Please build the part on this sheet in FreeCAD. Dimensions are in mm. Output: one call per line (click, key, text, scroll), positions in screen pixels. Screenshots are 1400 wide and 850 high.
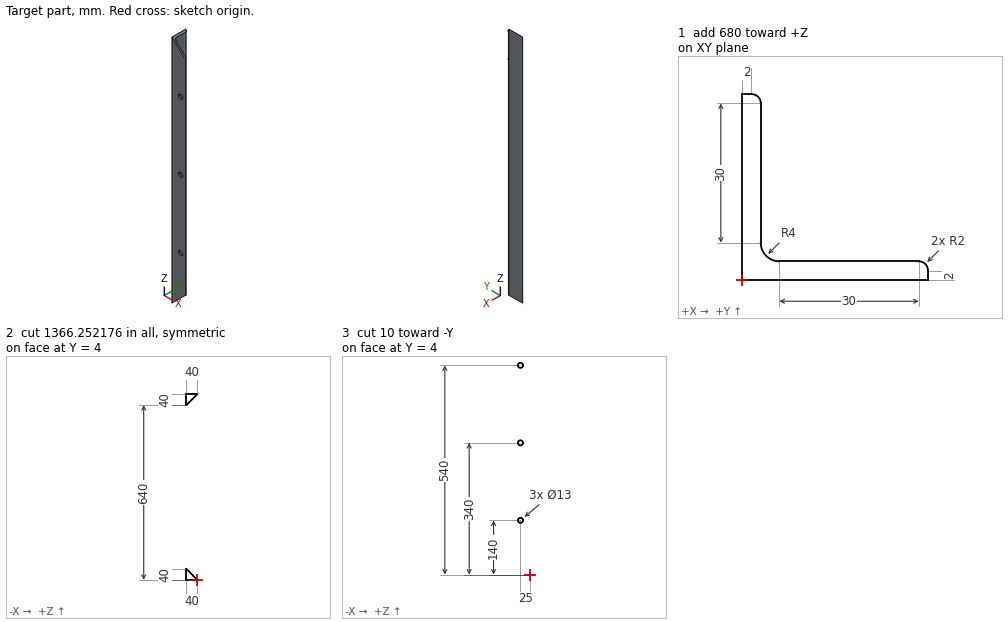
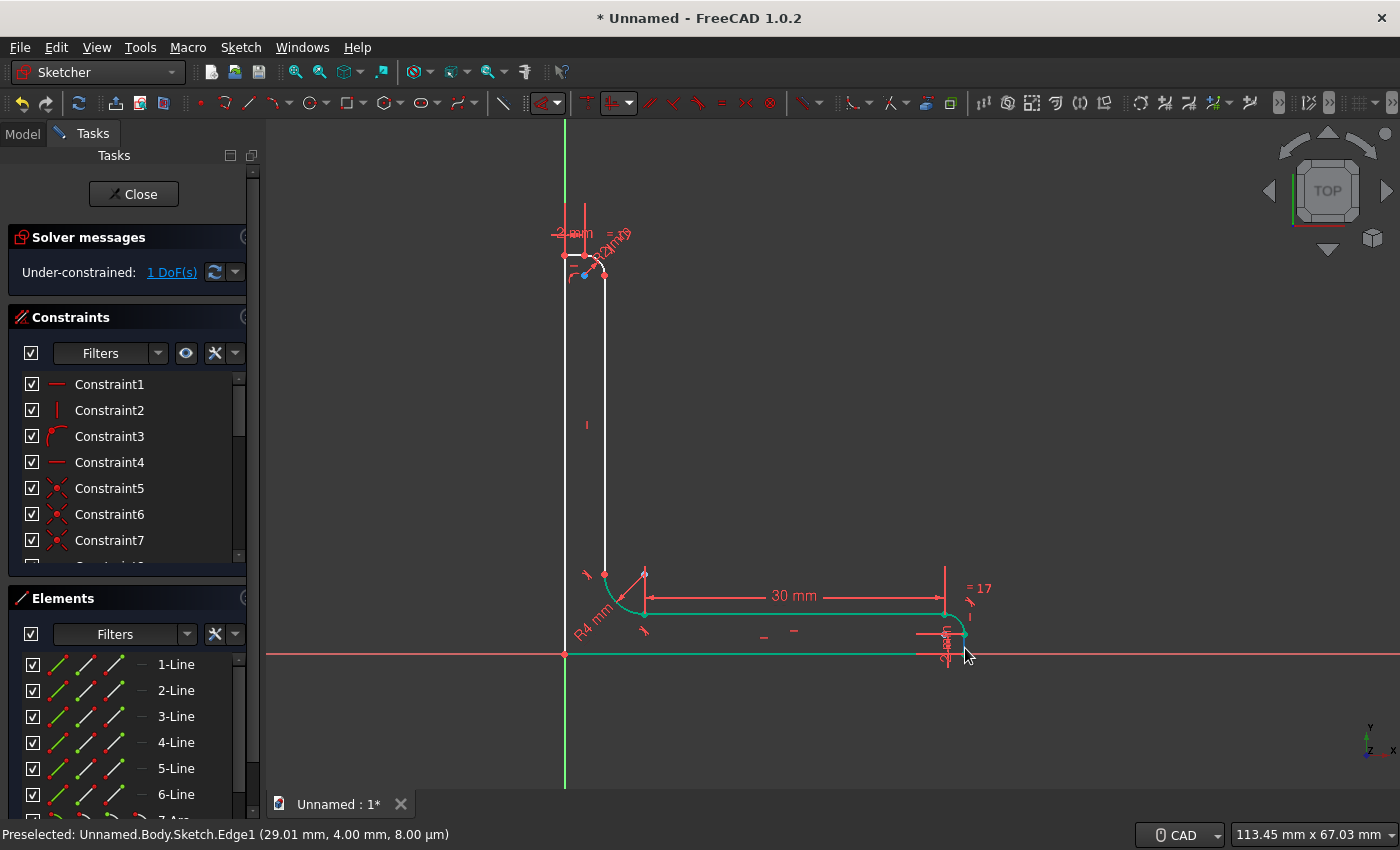
click(605, 484)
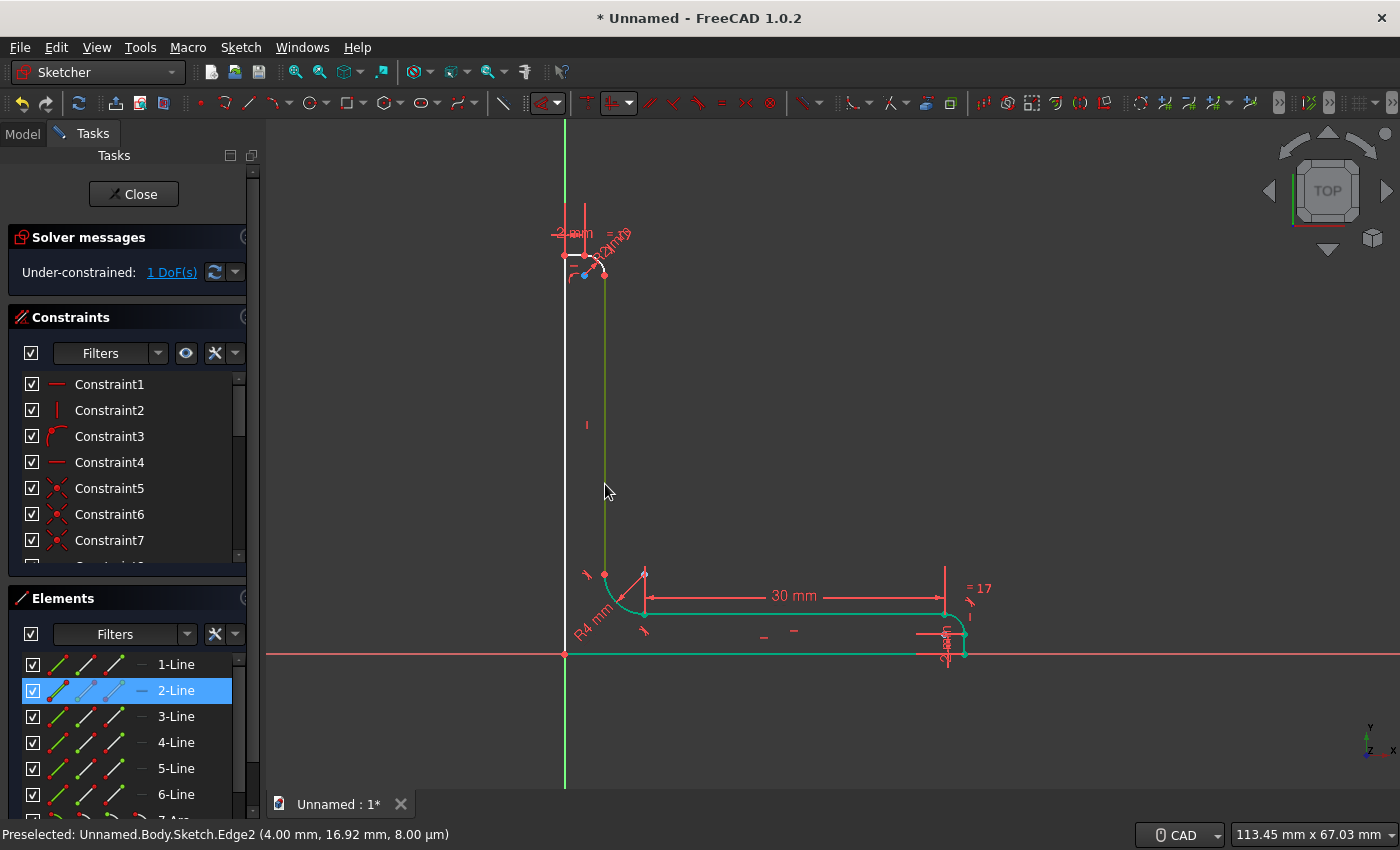
key(i)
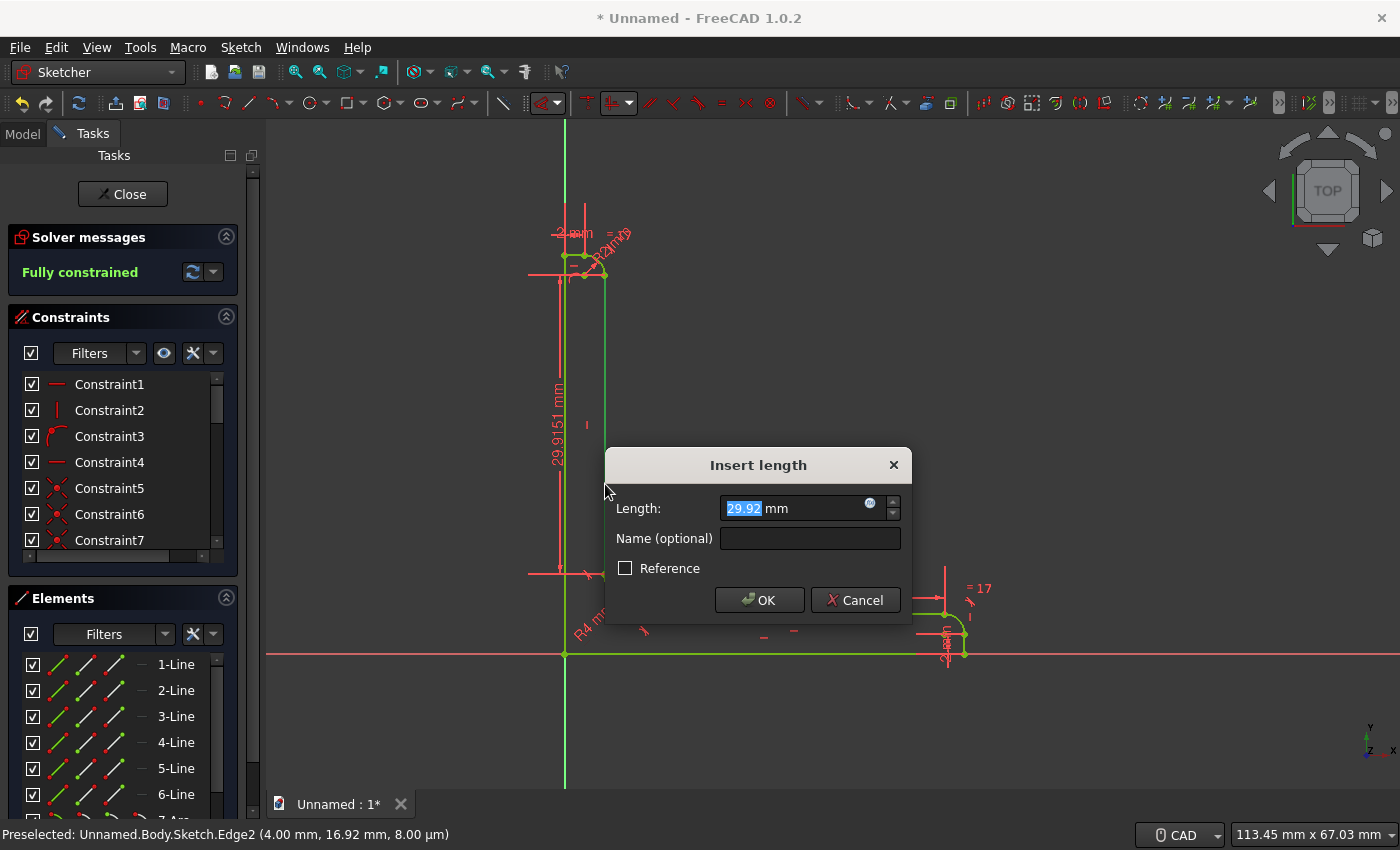
text(30)
key(Return)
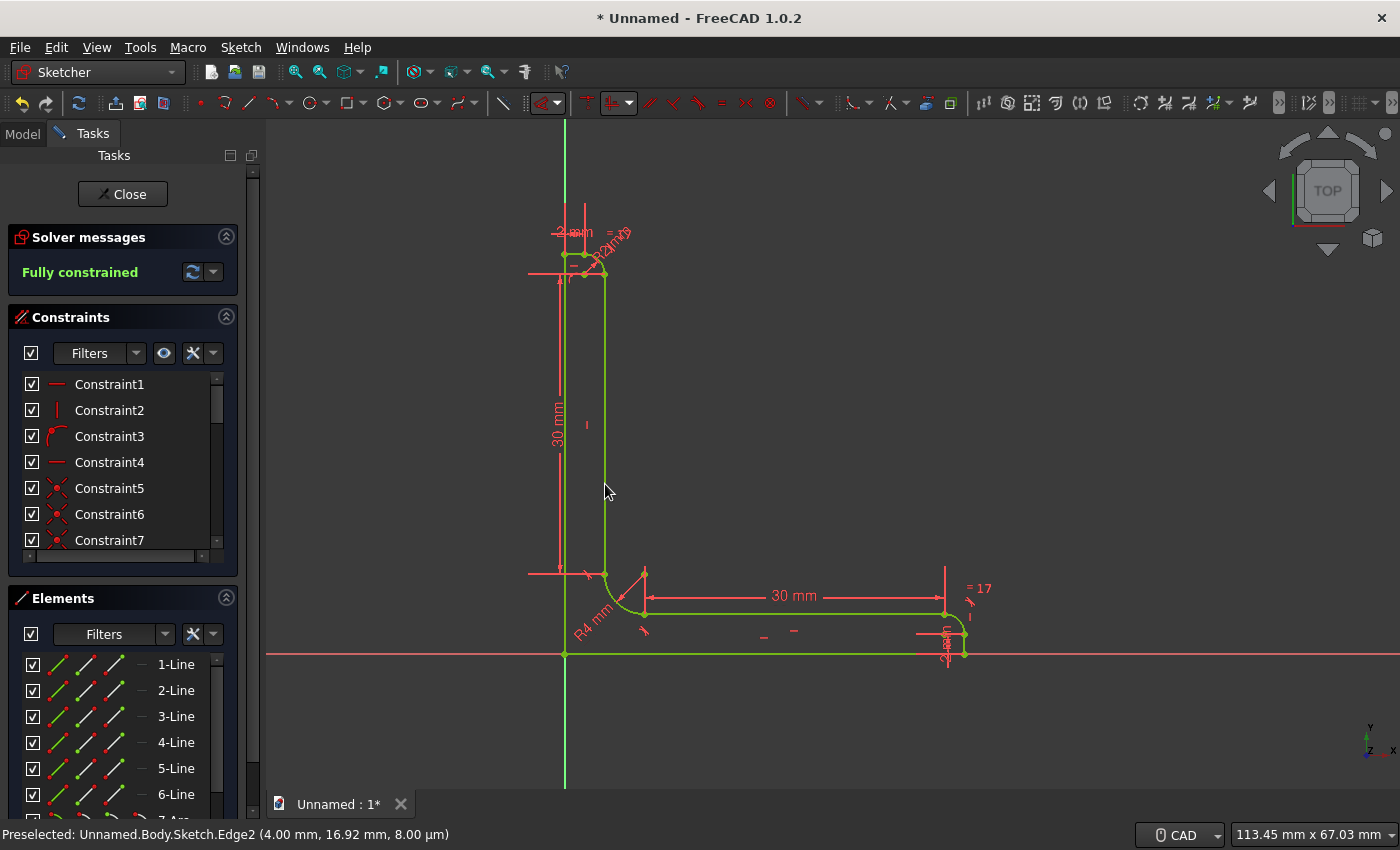
click(123, 194)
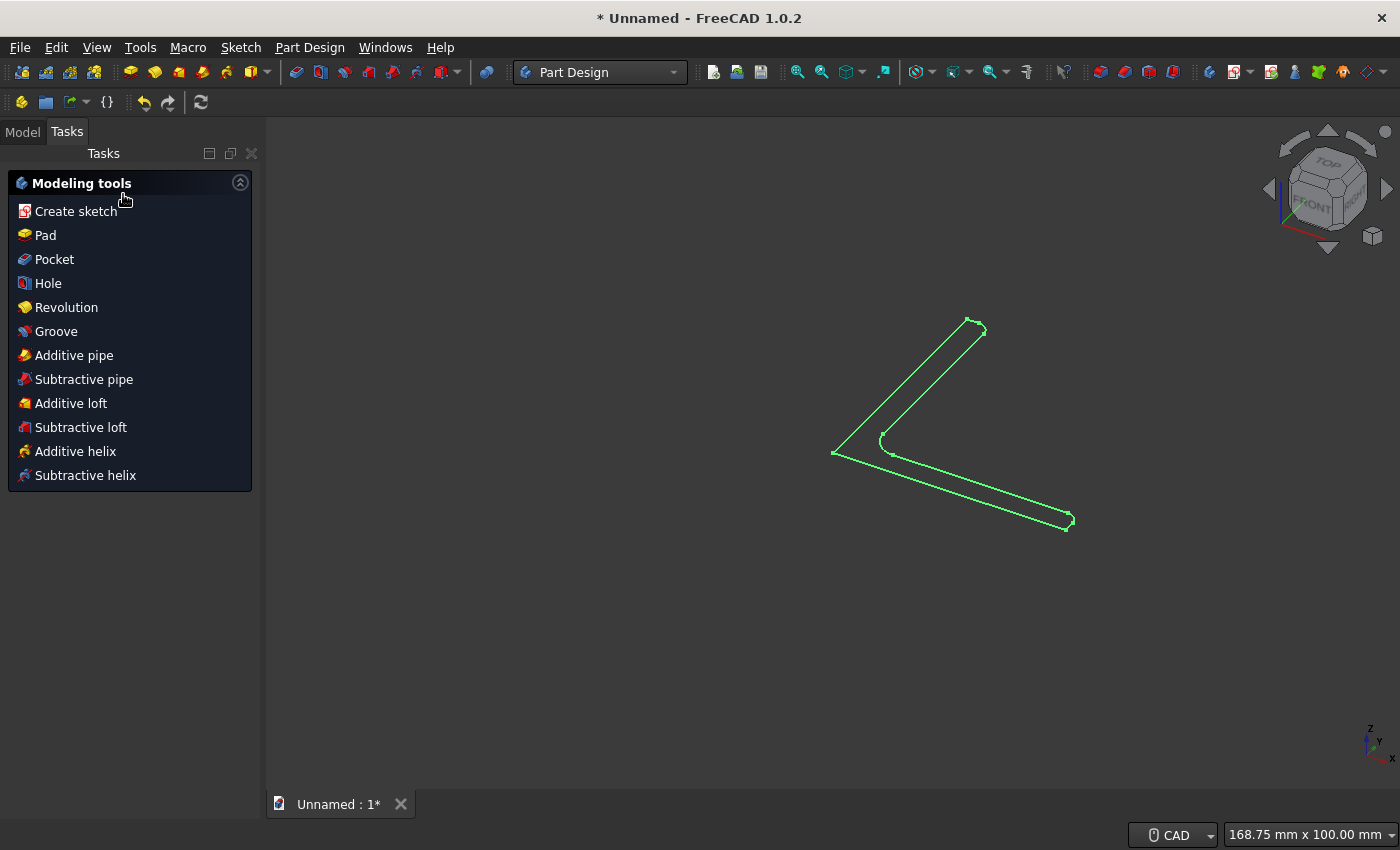
click(132, 72)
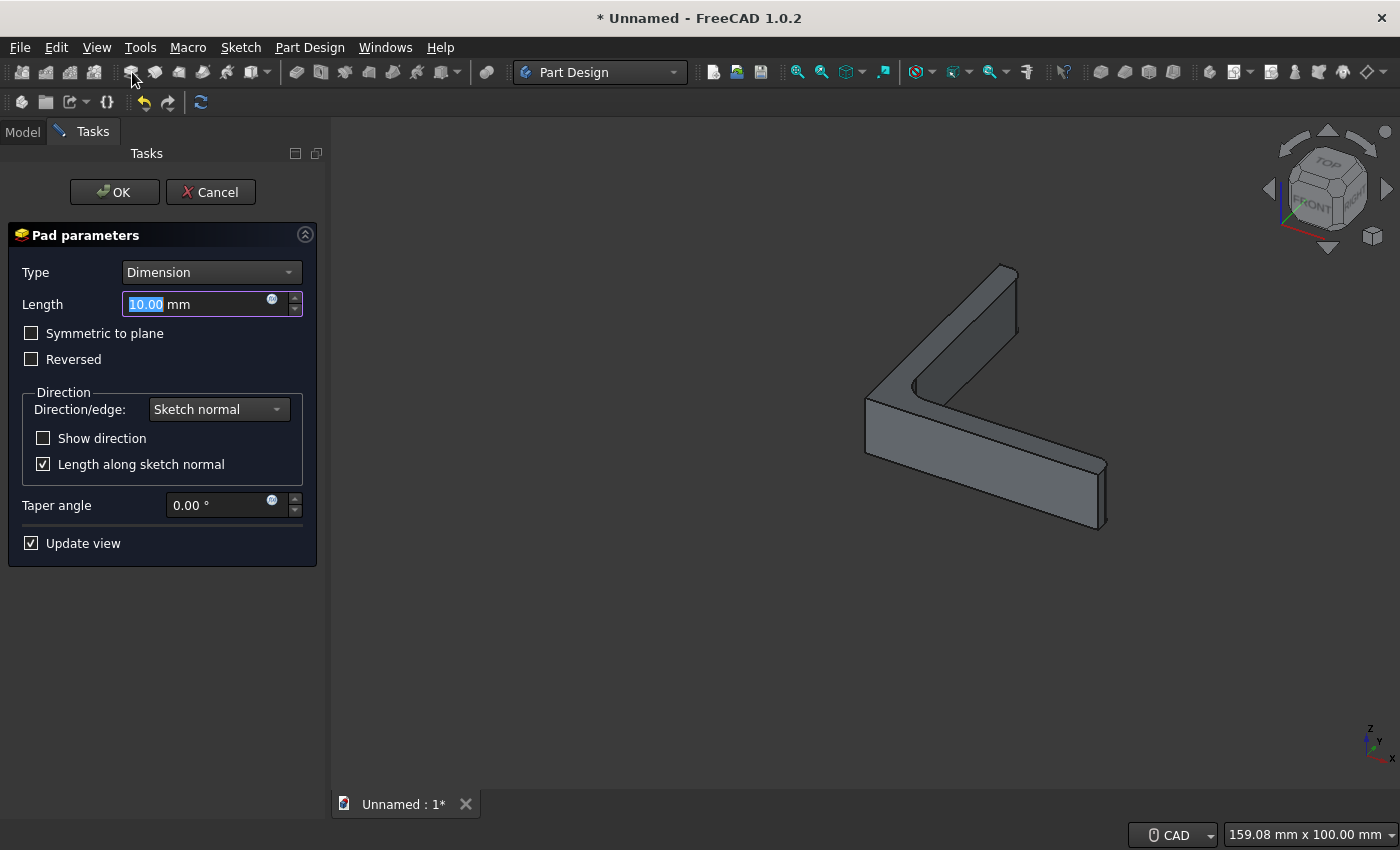
text(680)
key(Tab)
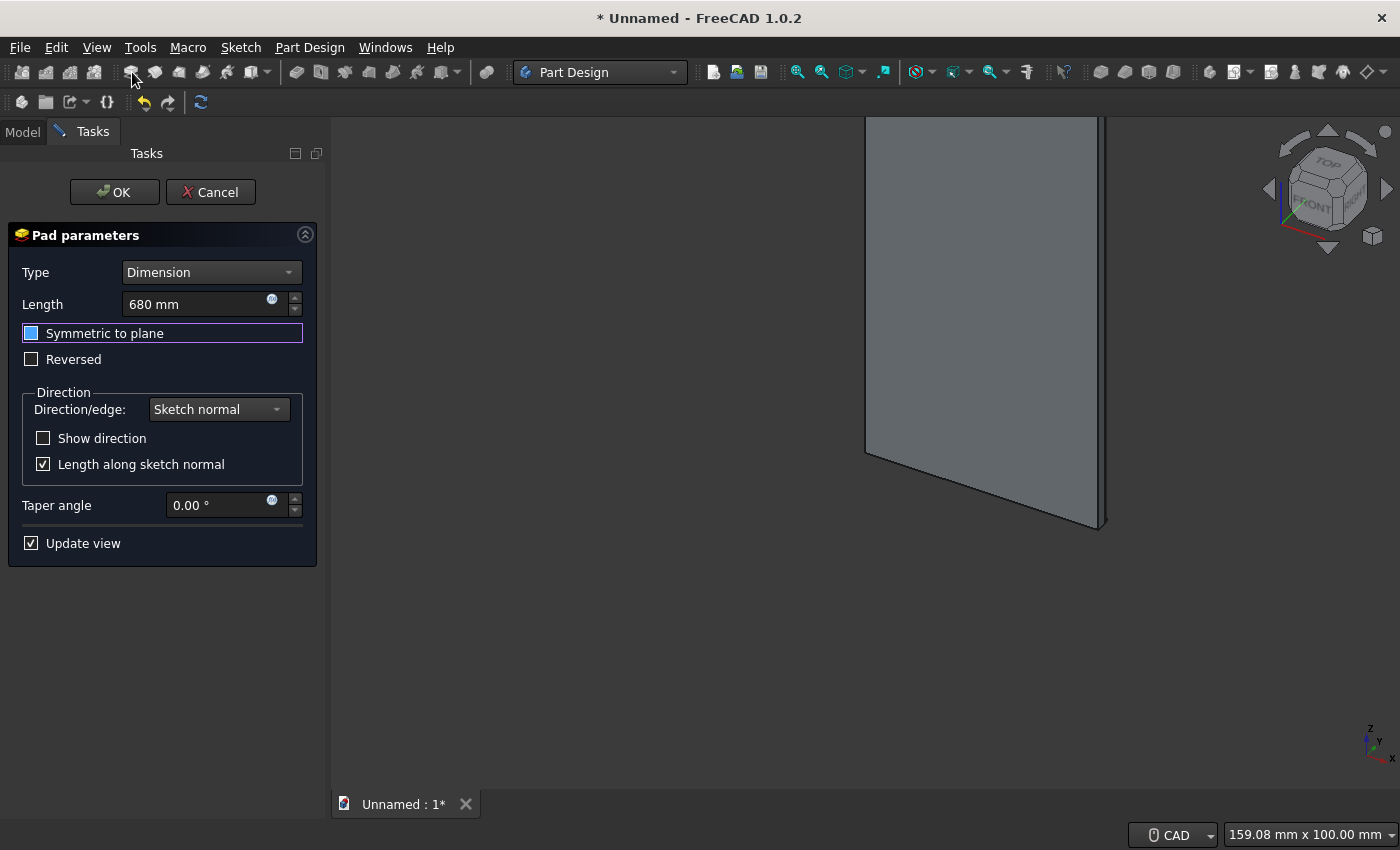
click(115, 192)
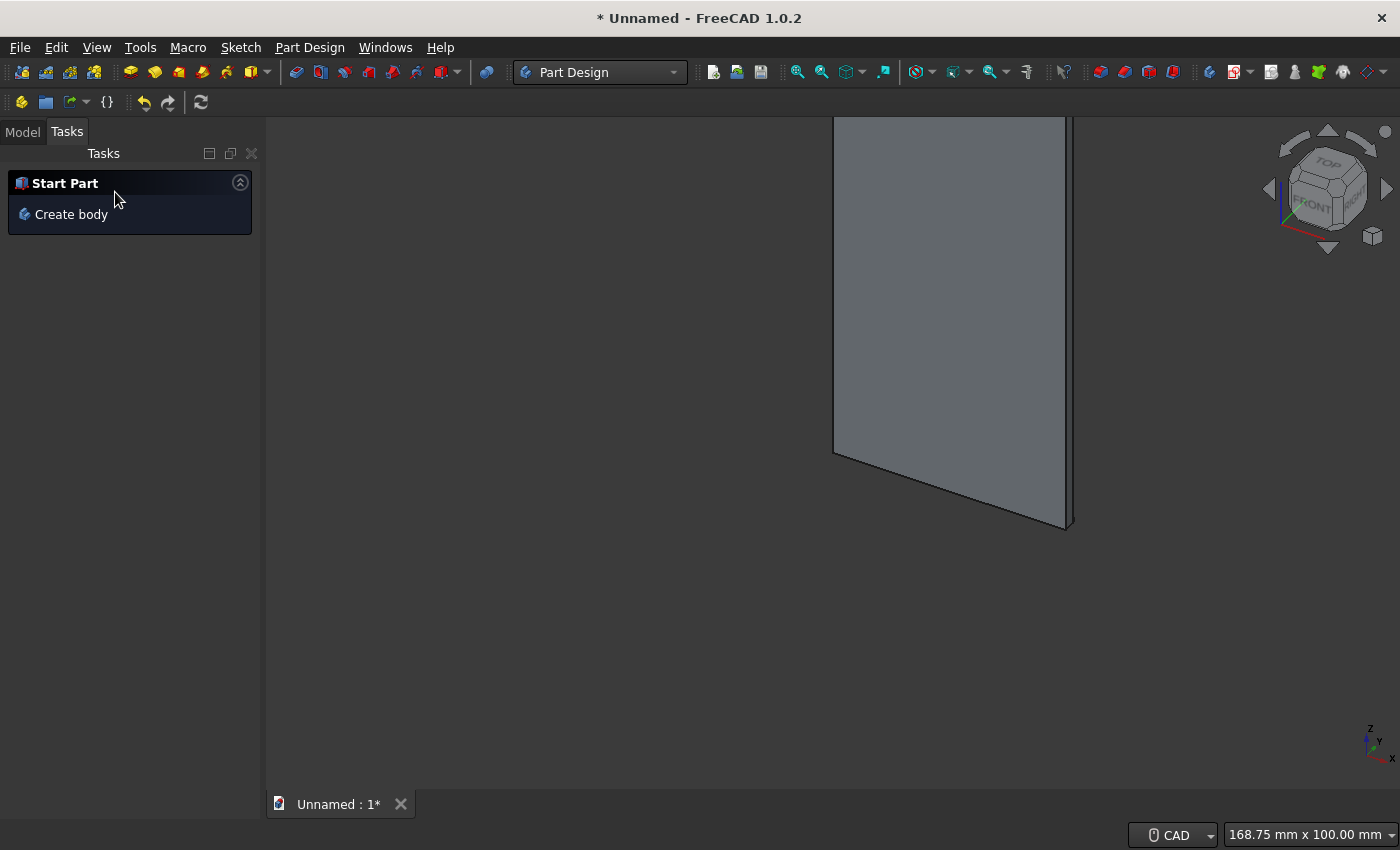
click(798, 72)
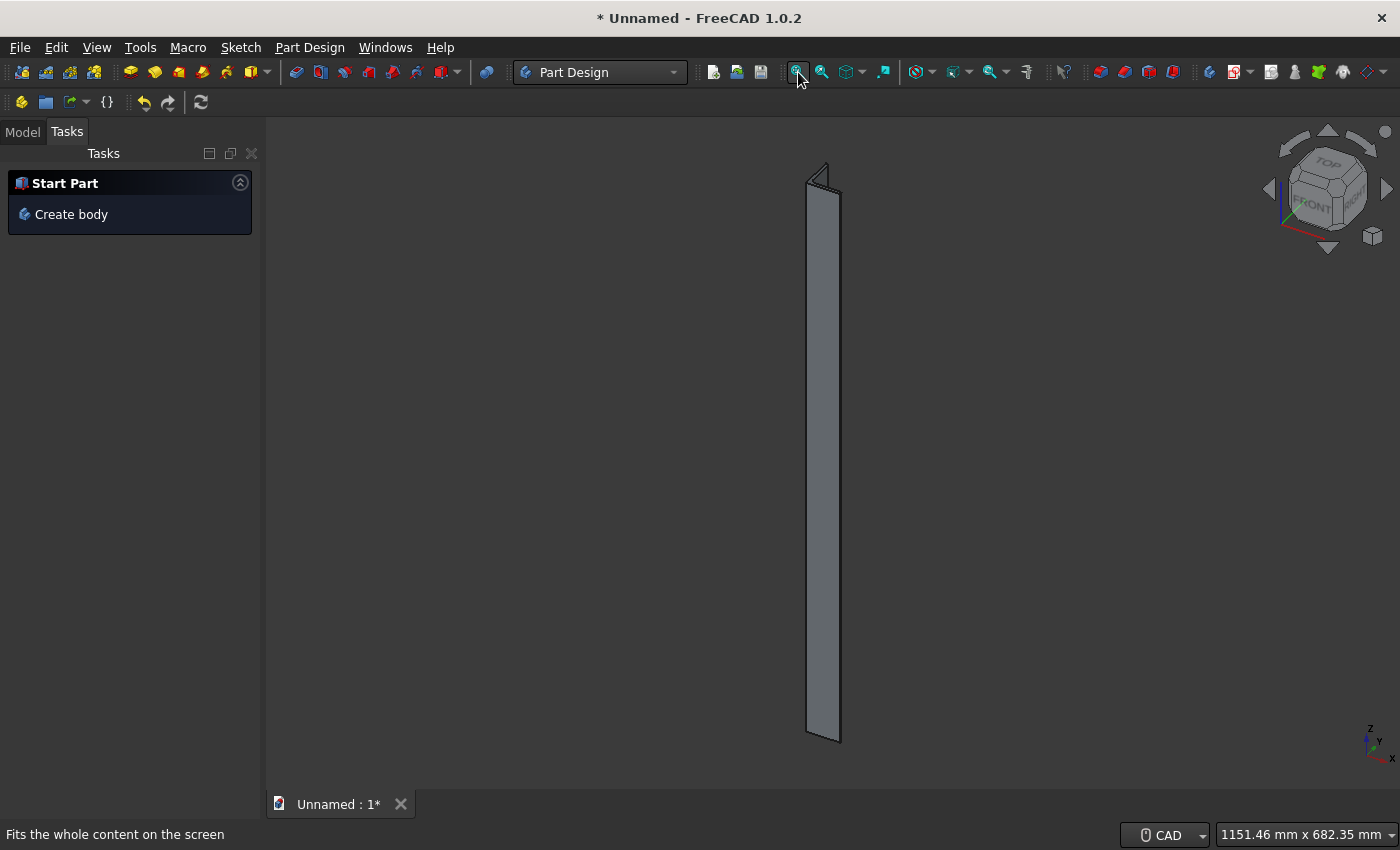
key(4)